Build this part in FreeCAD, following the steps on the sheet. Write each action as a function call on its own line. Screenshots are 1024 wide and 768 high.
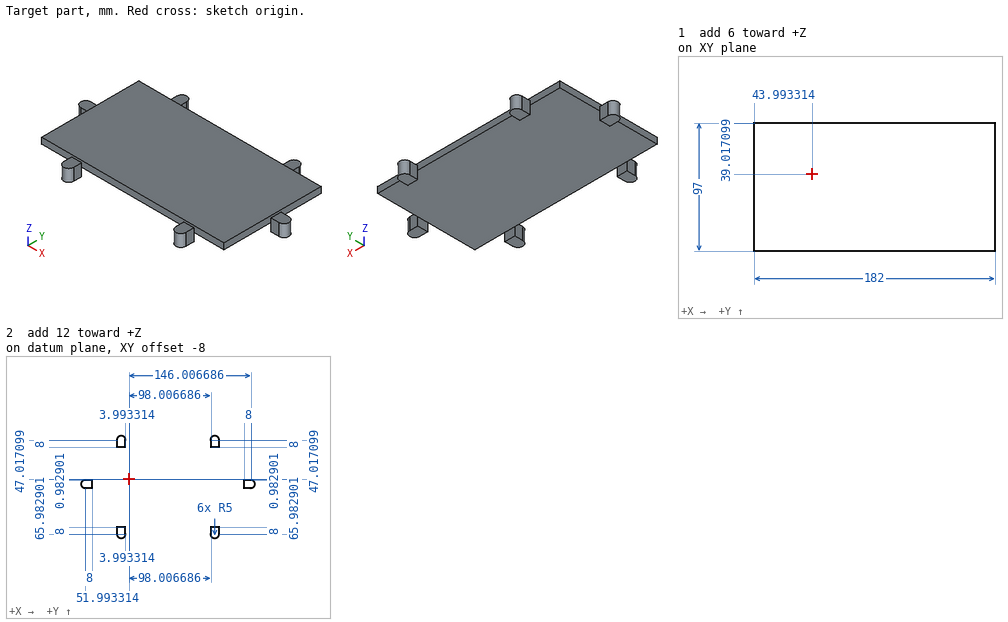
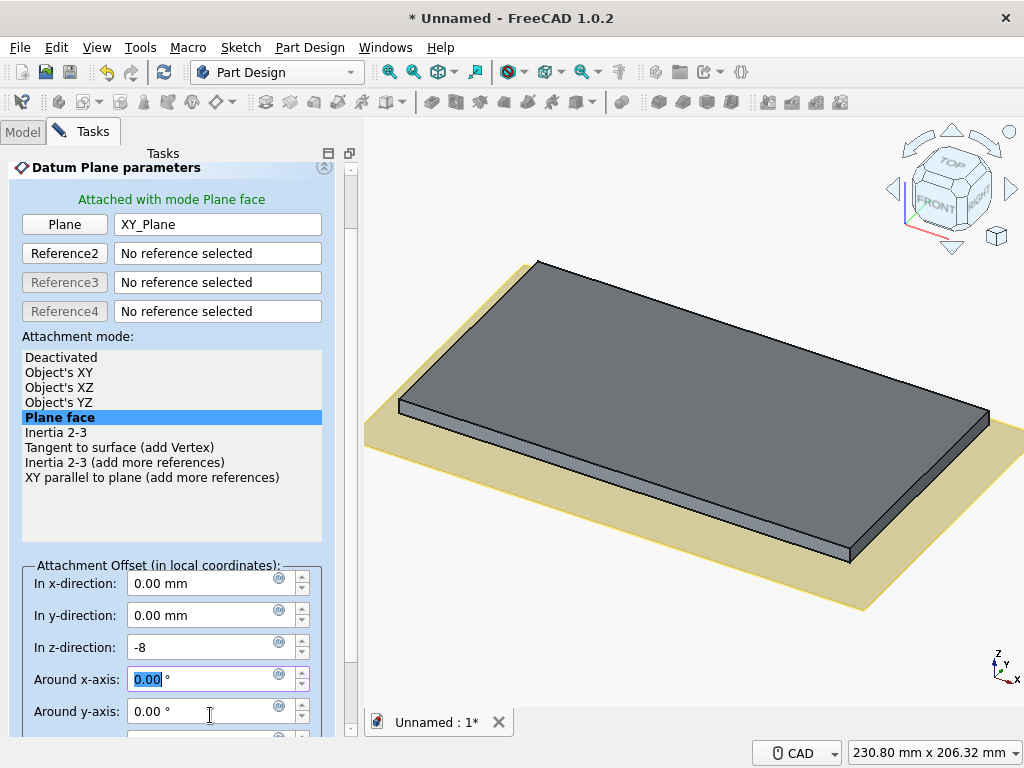
scroll(351, 450, up, 2)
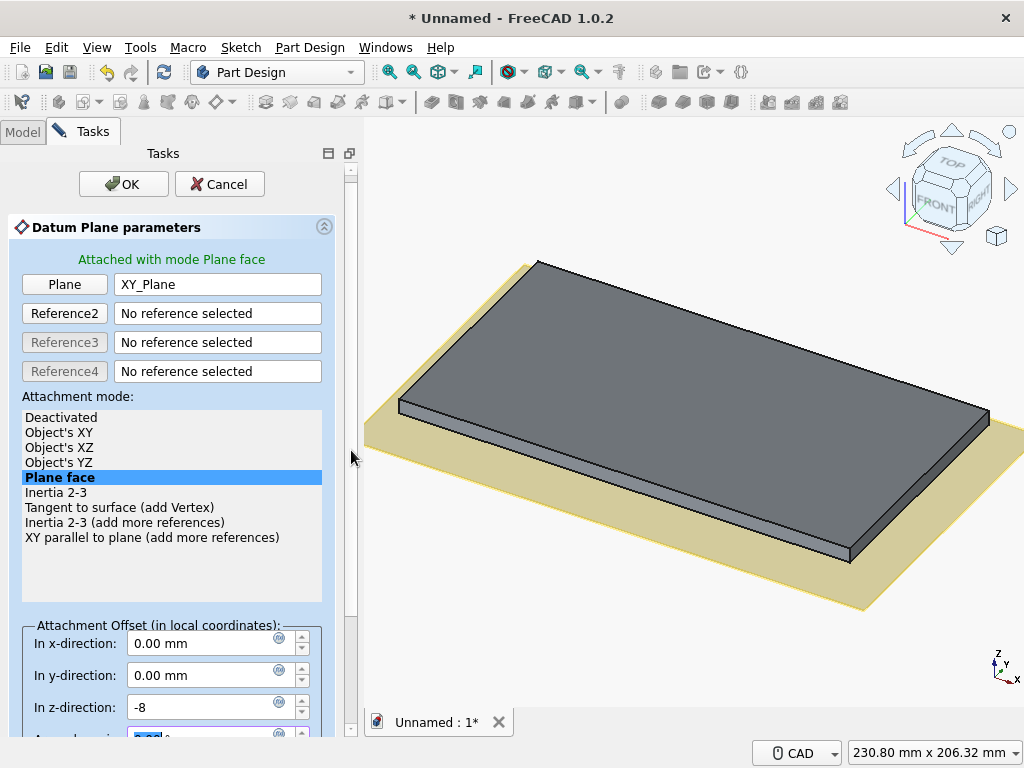
click(124, 192)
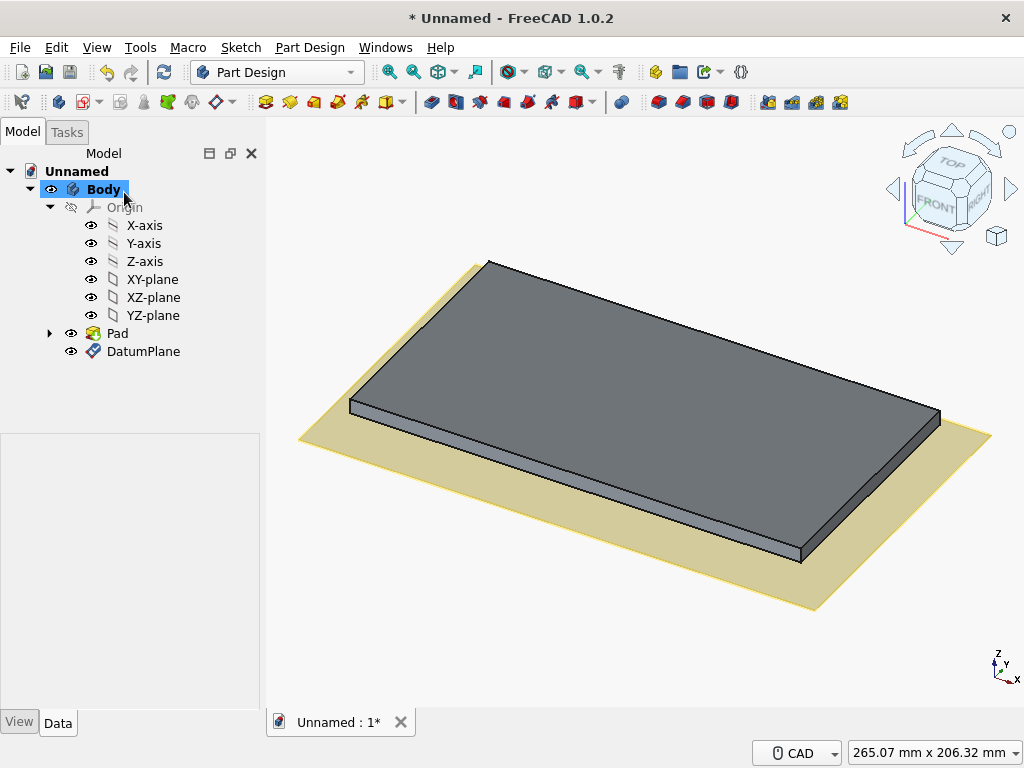
click(116, 351)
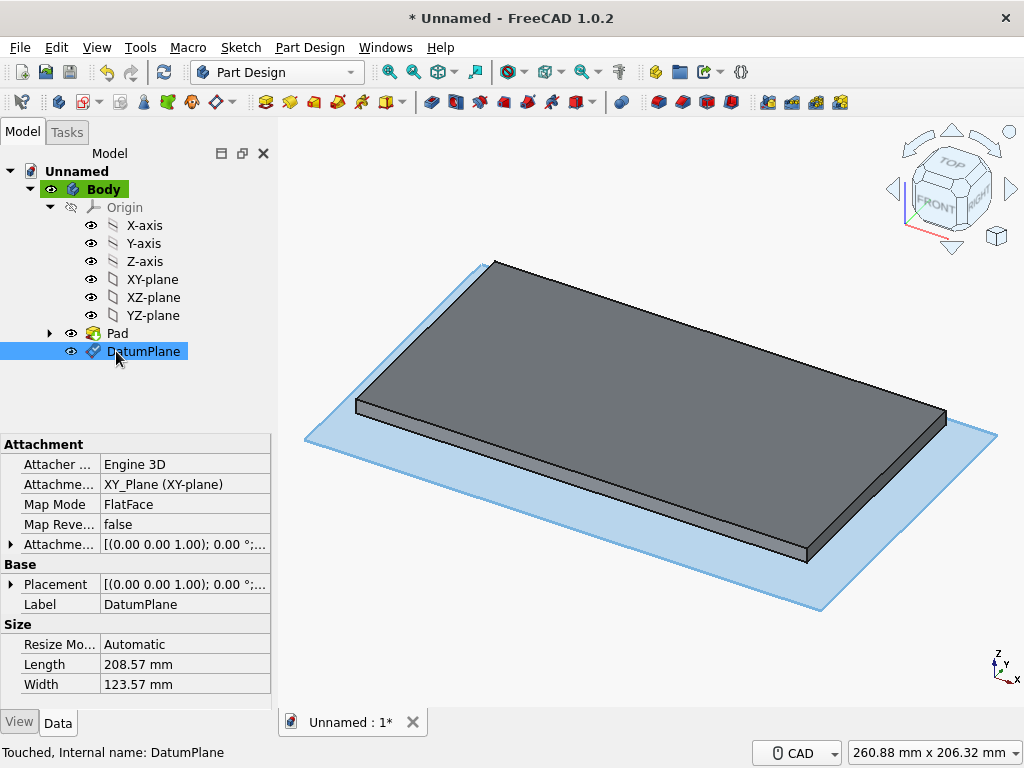
click(84, 102)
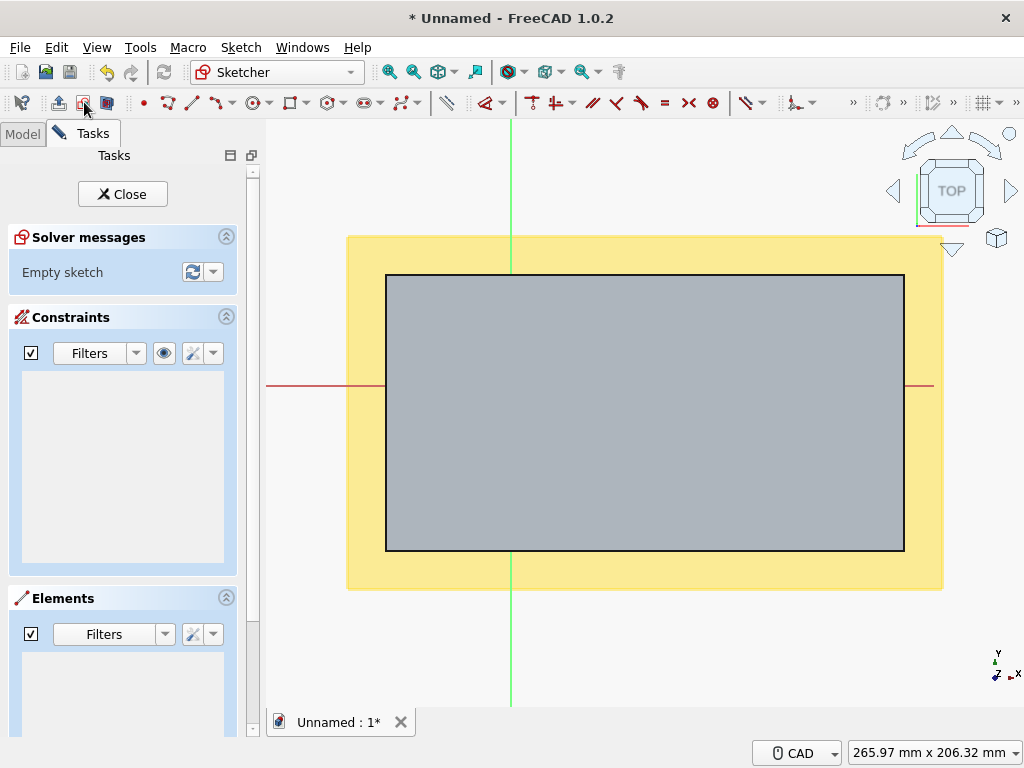
click(108, 104)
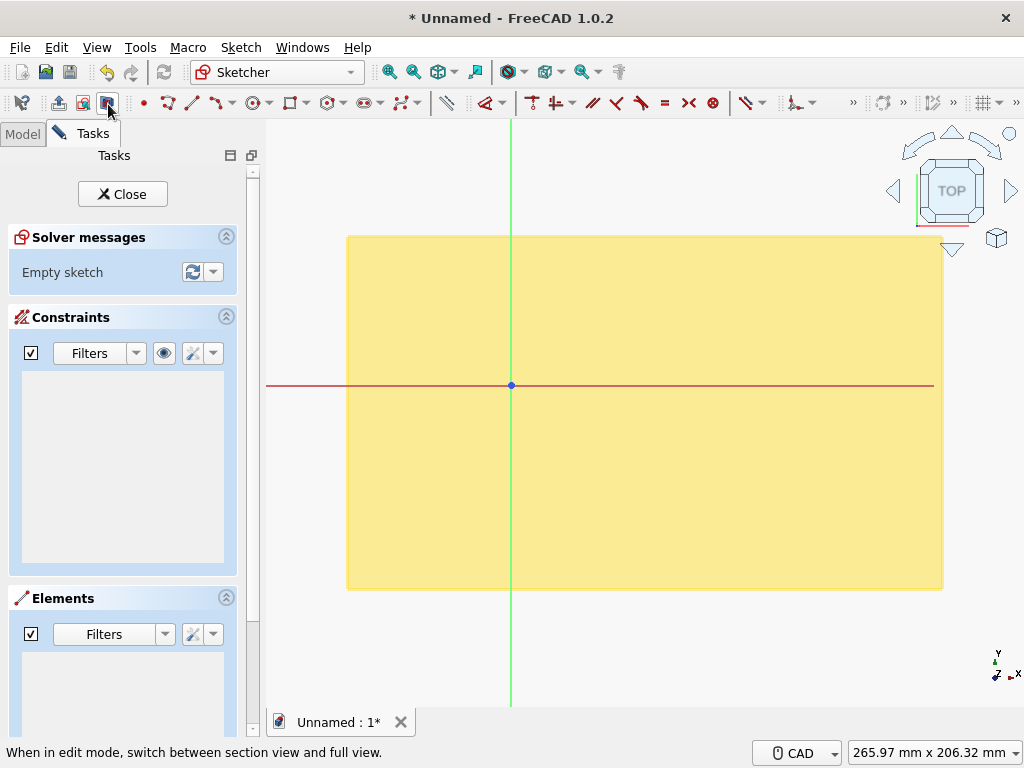
scroll(437, 413, down, 2)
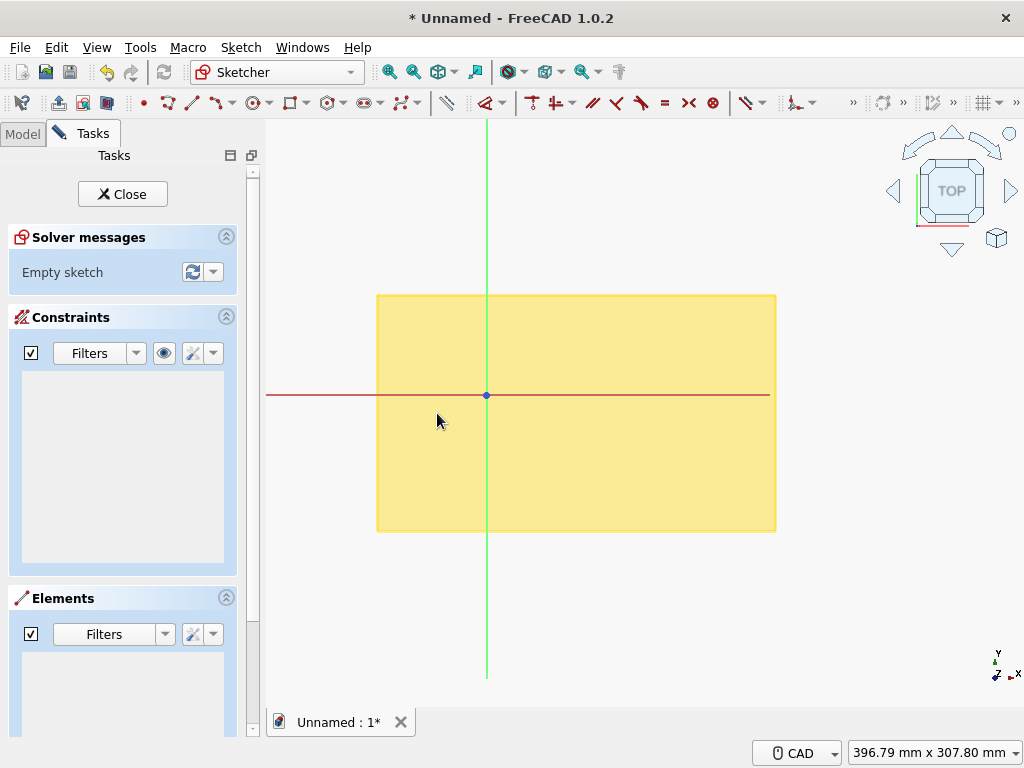
click(168, 104)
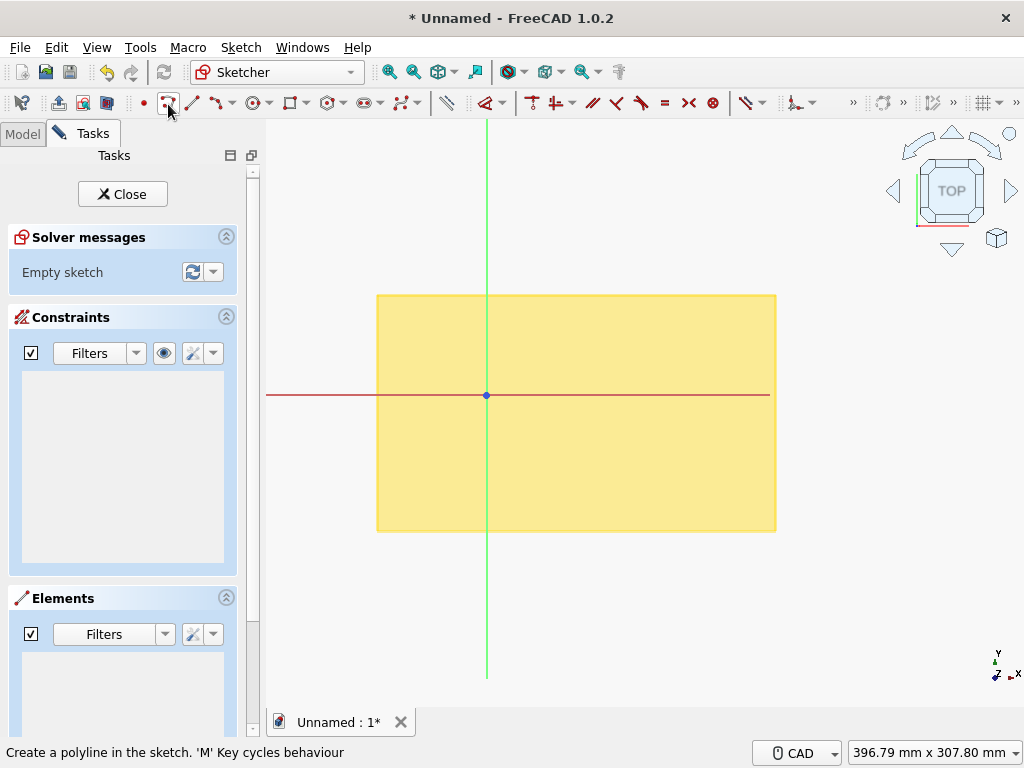
click(693, 521)
click(693, 506)
click(674, 506)
click(674, 521)
right_click(674, 521)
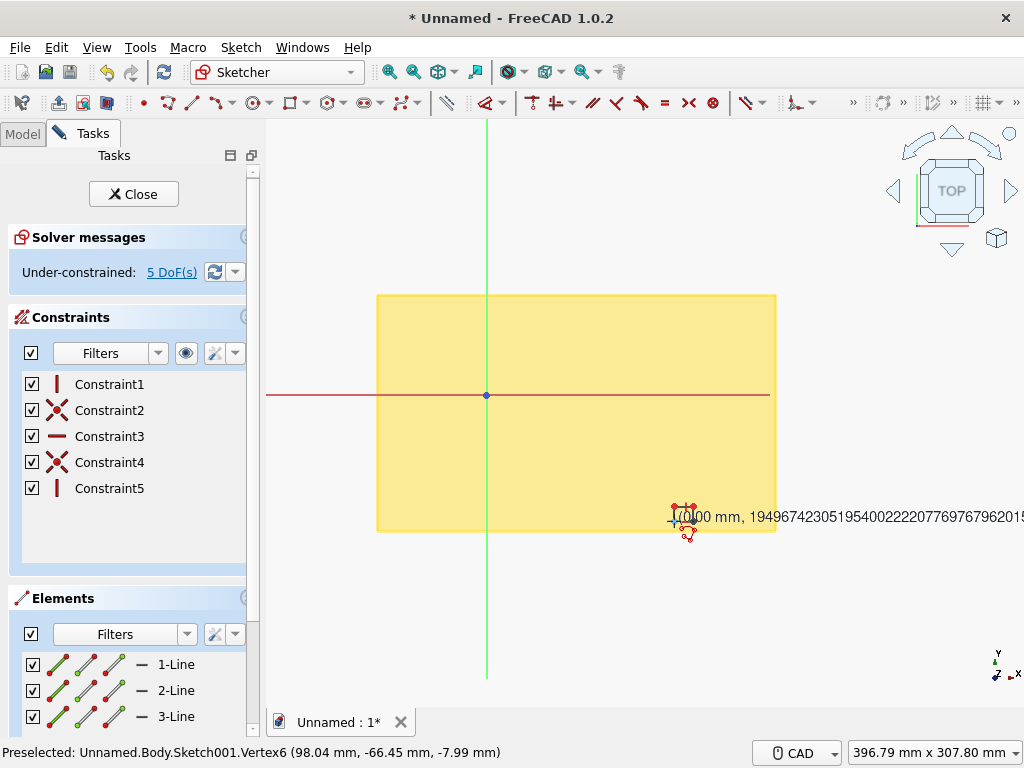
click(216, 104)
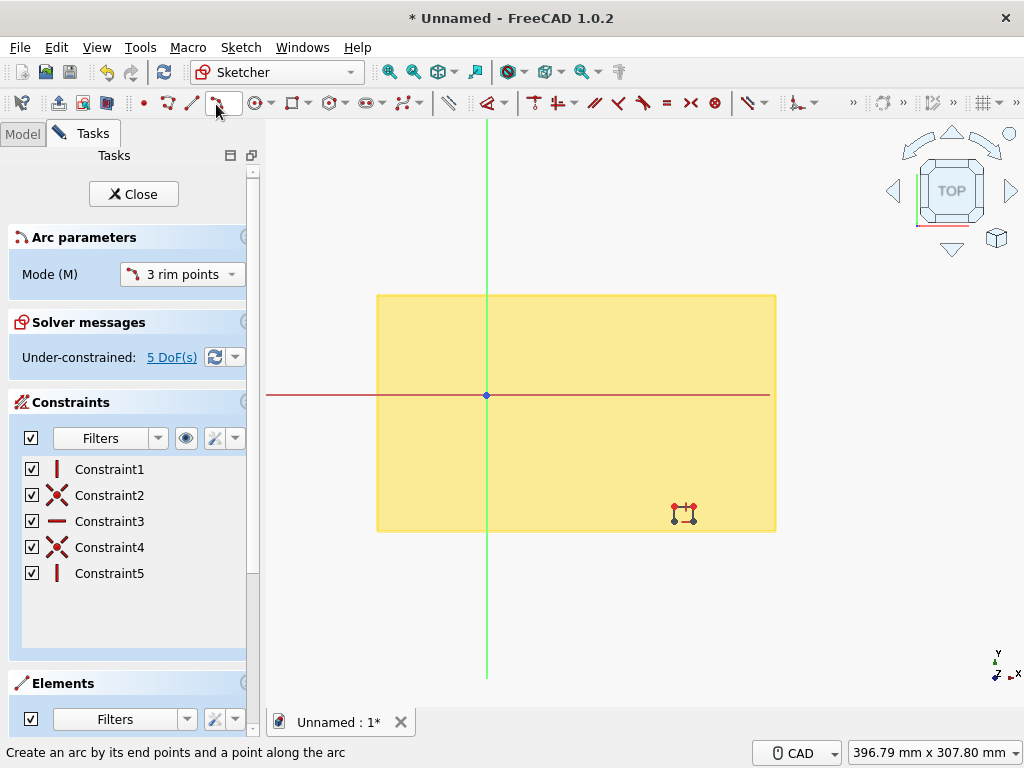
scroll(674, 521, up, 4)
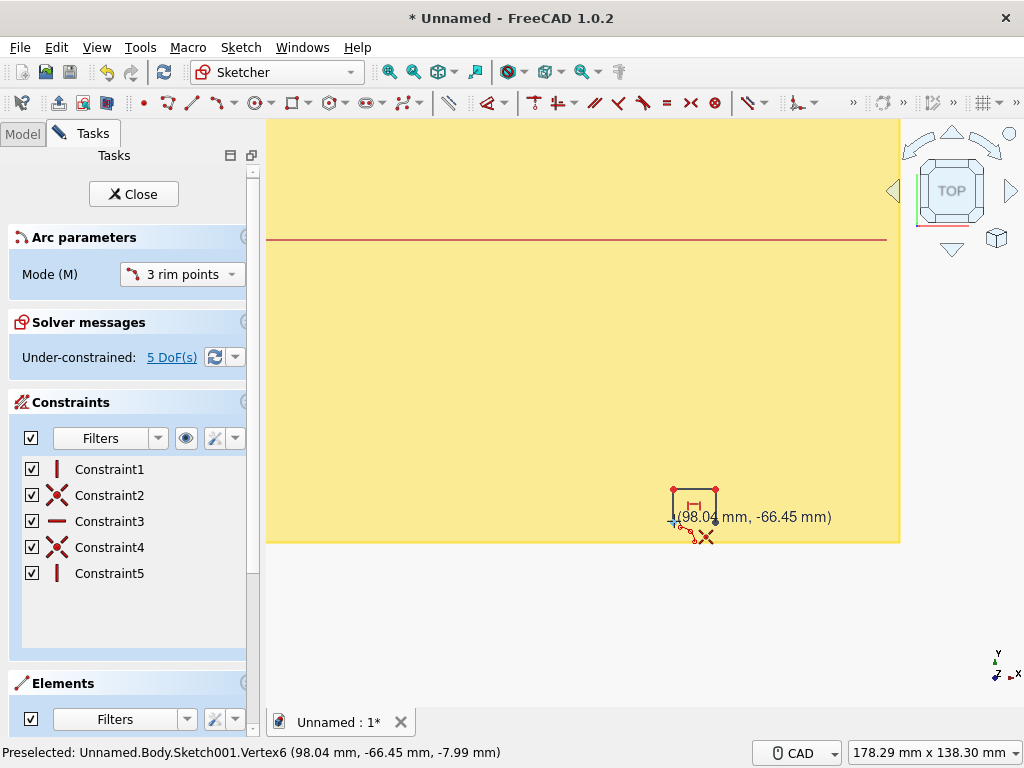
click(673, 522)
click(716, 522)
click(694, 542)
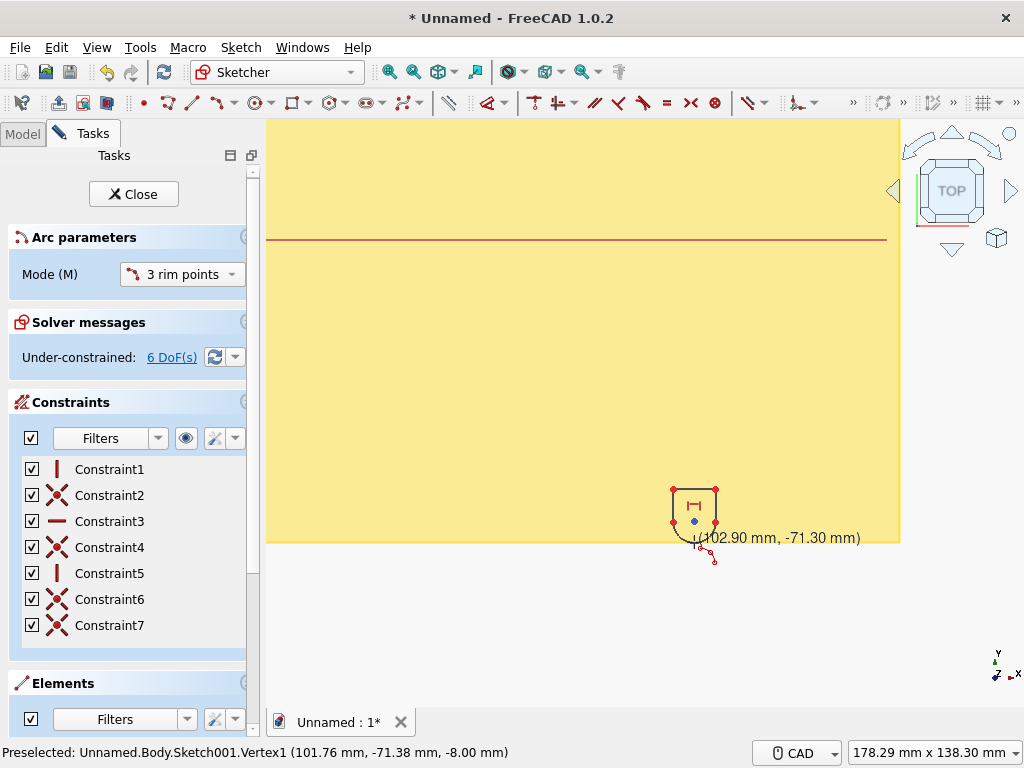
click(168, 104)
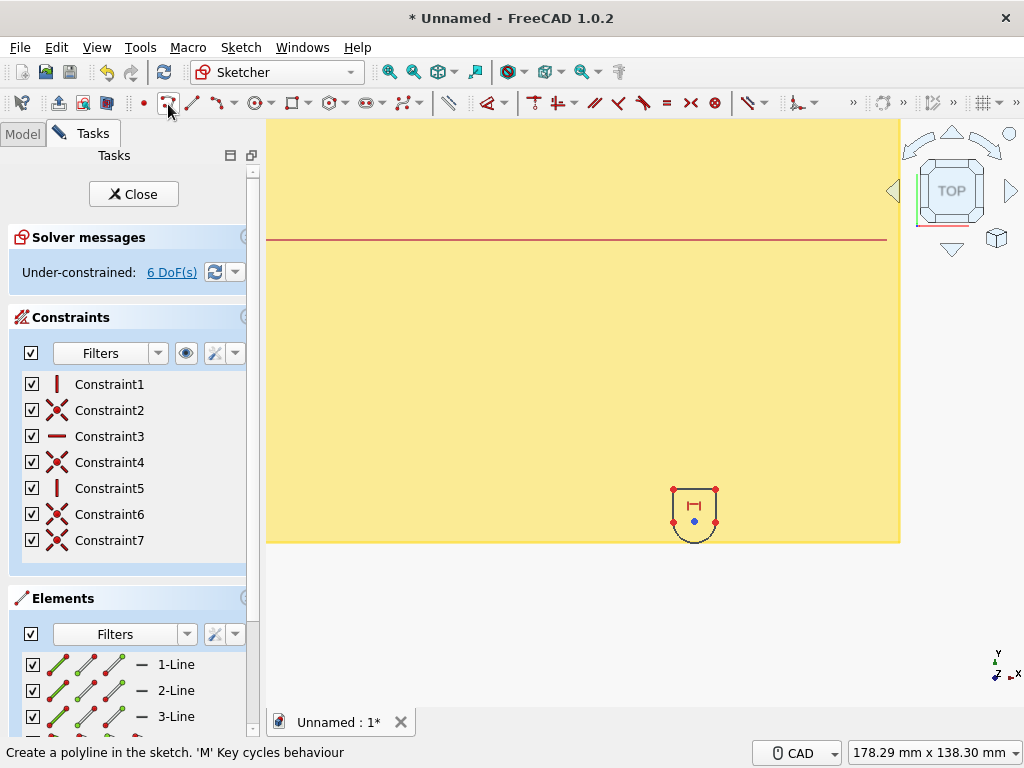
scroll(675, 521, down, 4)